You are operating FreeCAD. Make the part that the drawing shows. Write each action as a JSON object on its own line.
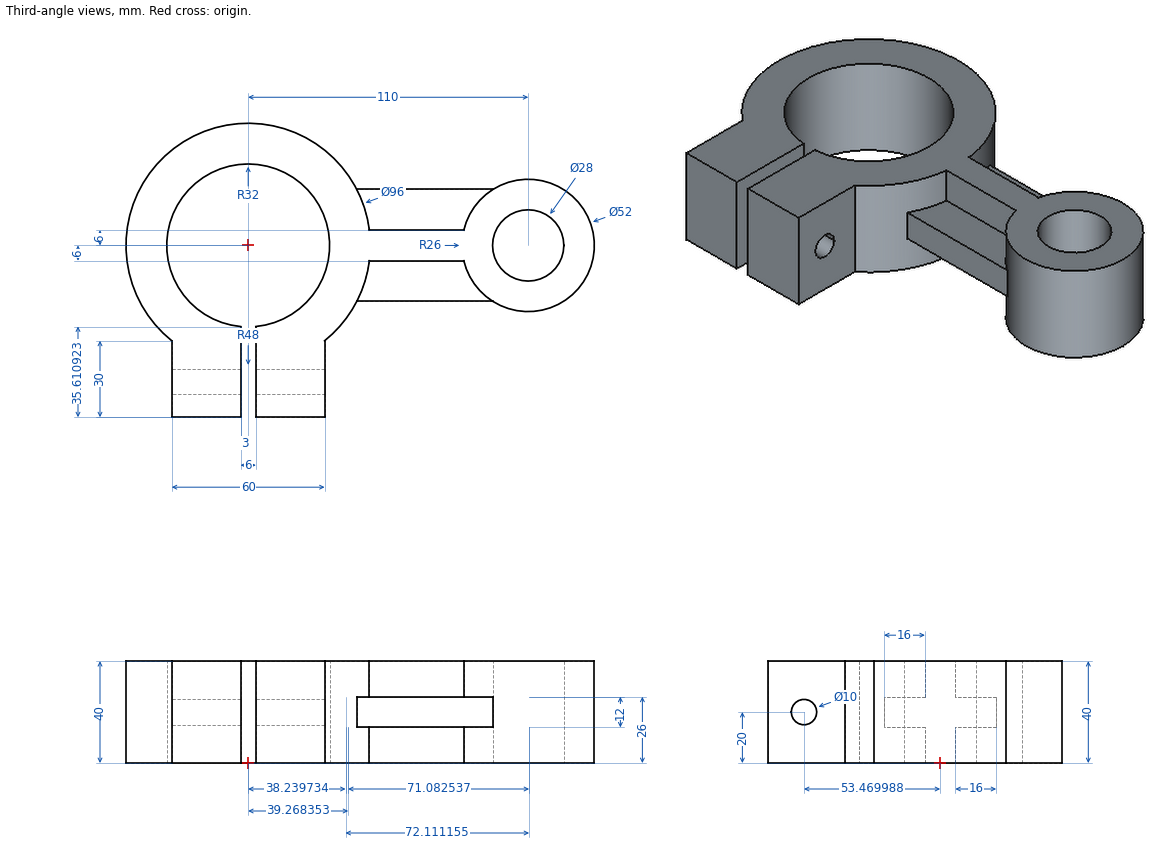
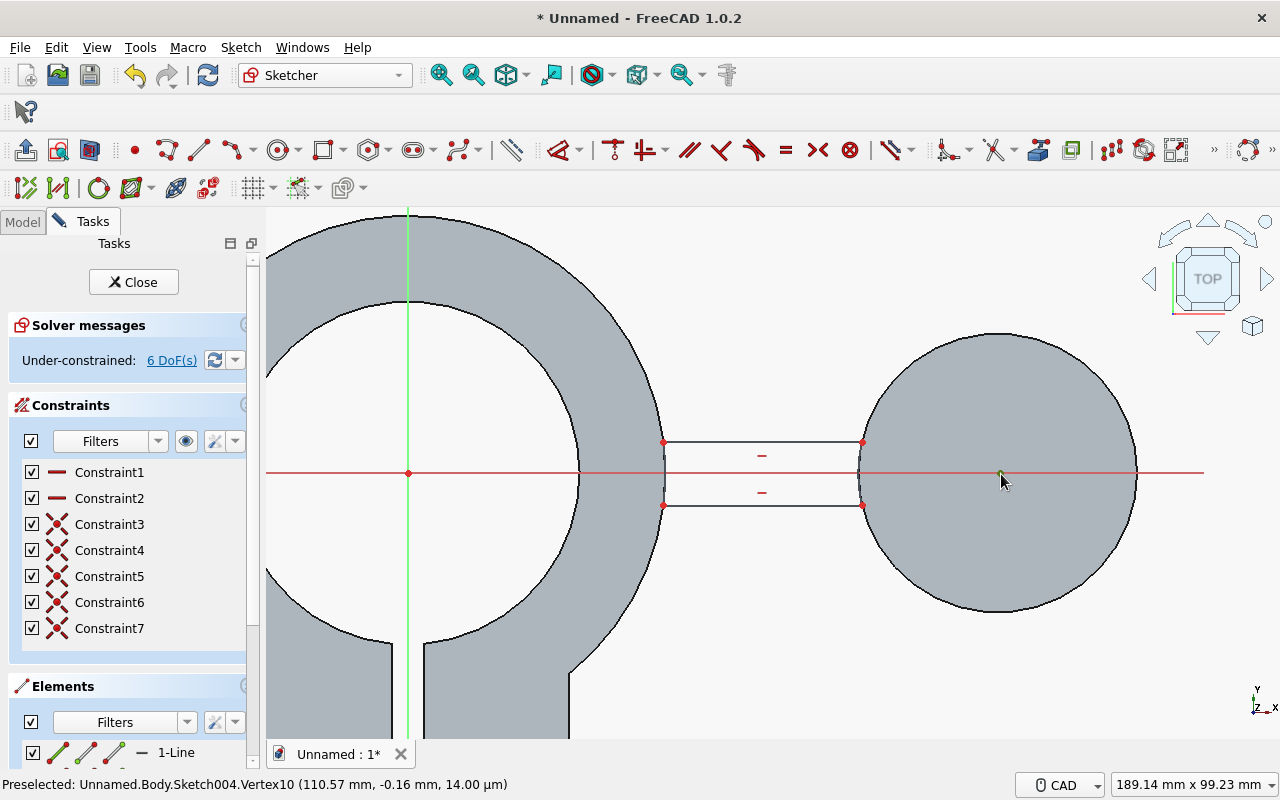
{"action": "left_click", "coordinate": [353, 473]}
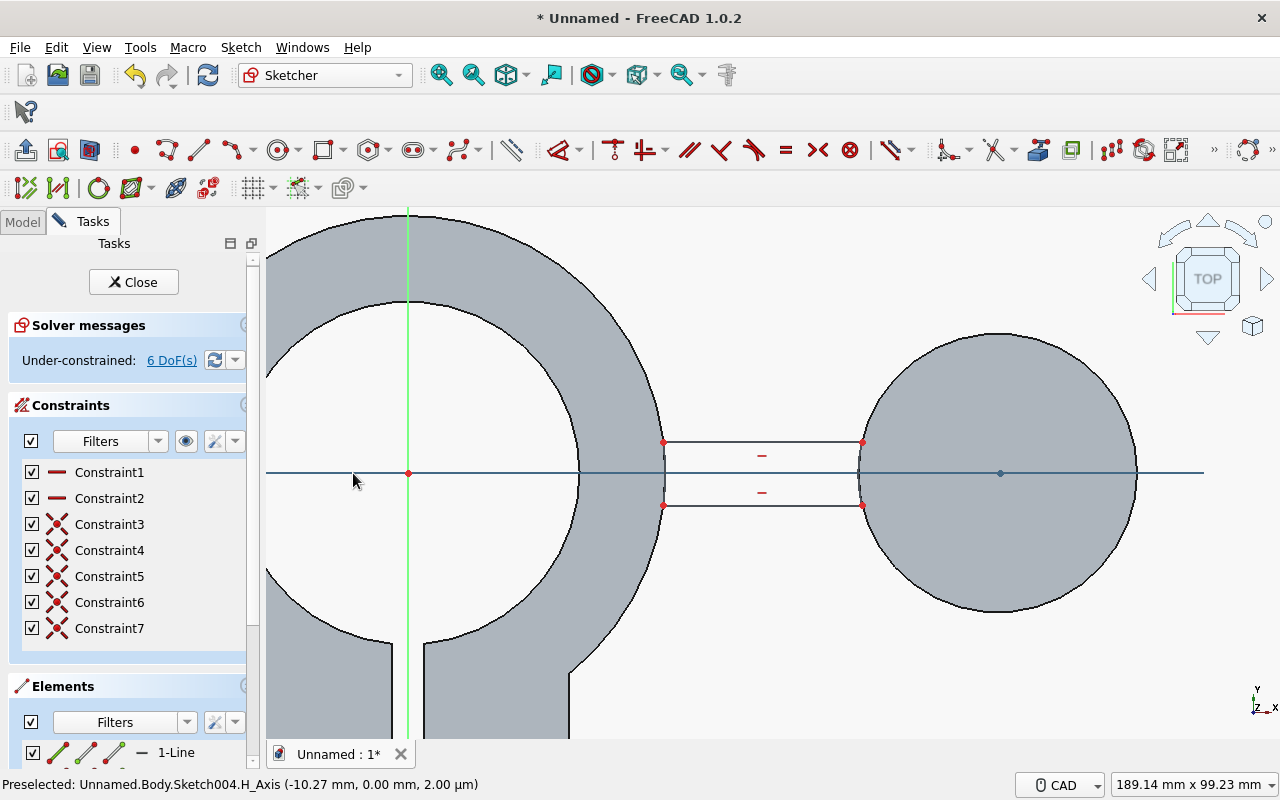
{"action": "left_click", "coordinate": [614, 150]}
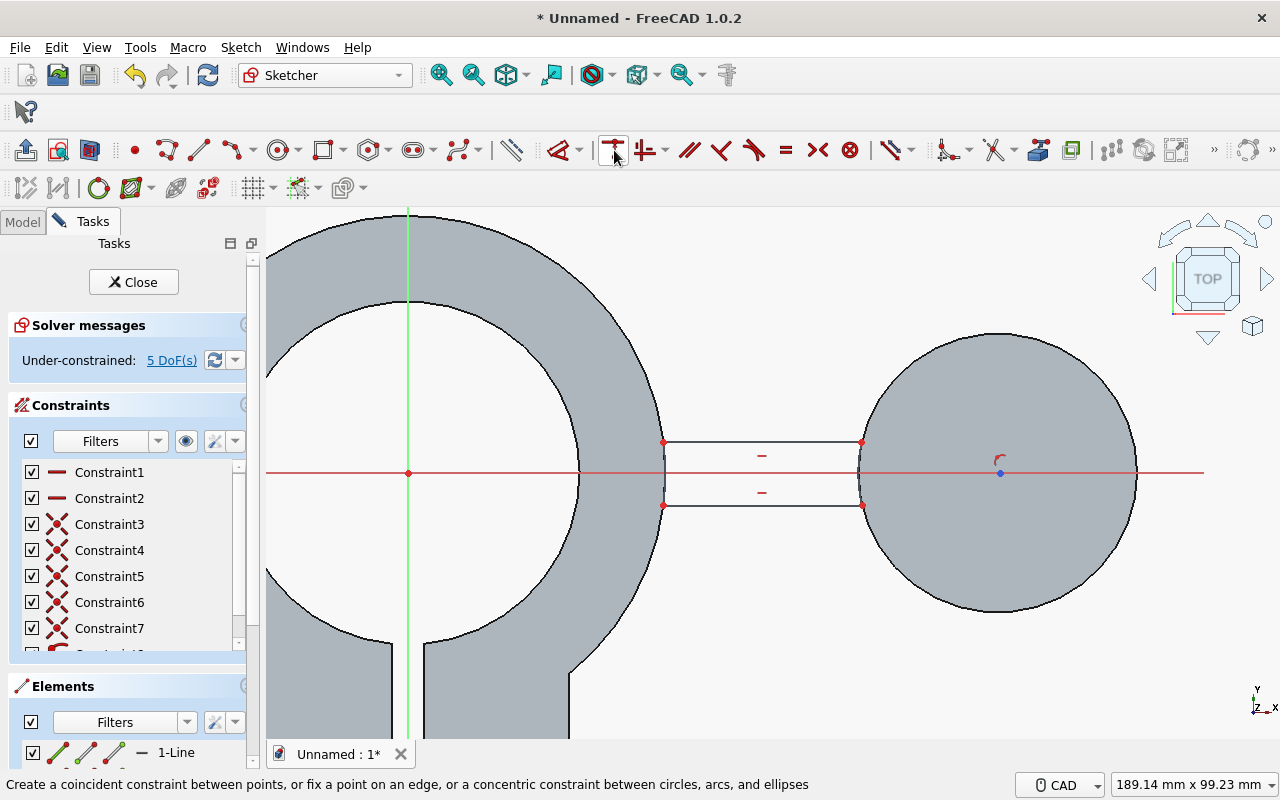
{"action": "left_click", "coordinate": [558, 150]}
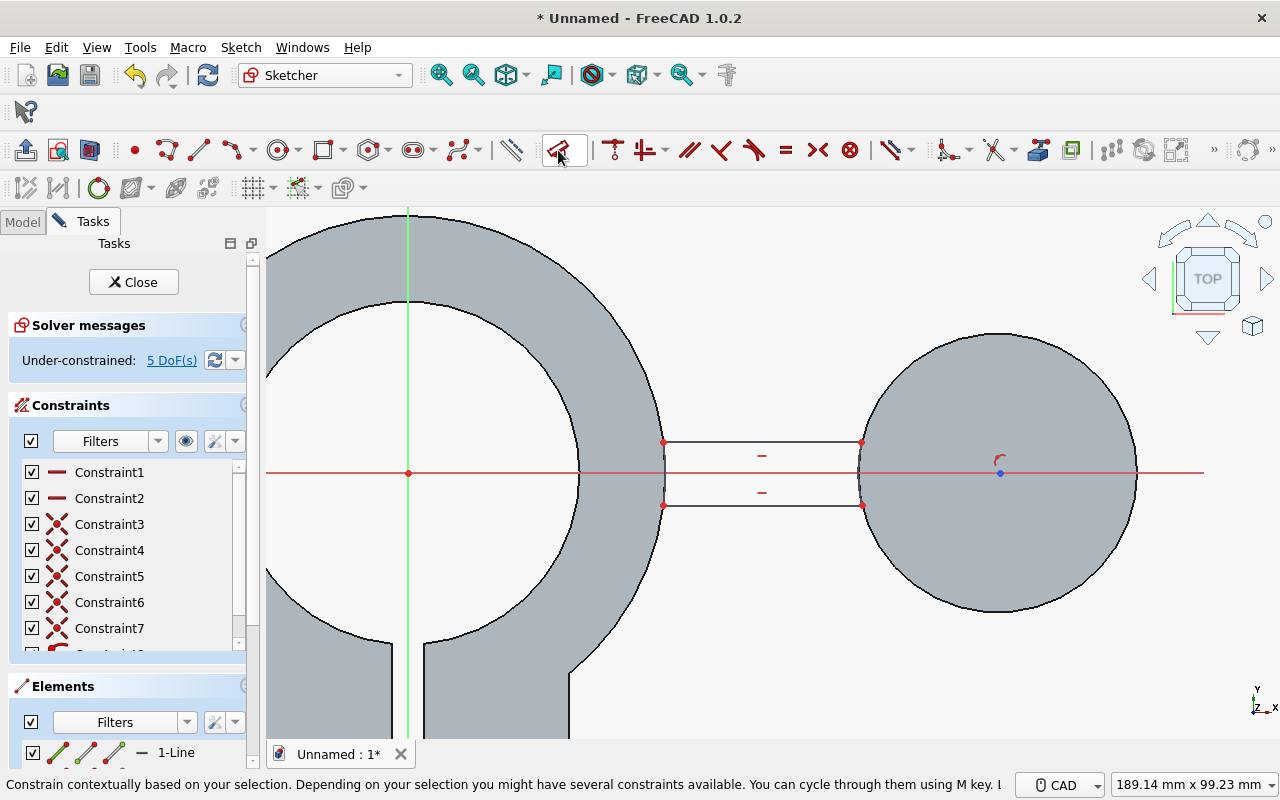
{"action": "left_click", "coordinate": [665, 487]}
{"action": "left_click", "coordinate": [697, 489]}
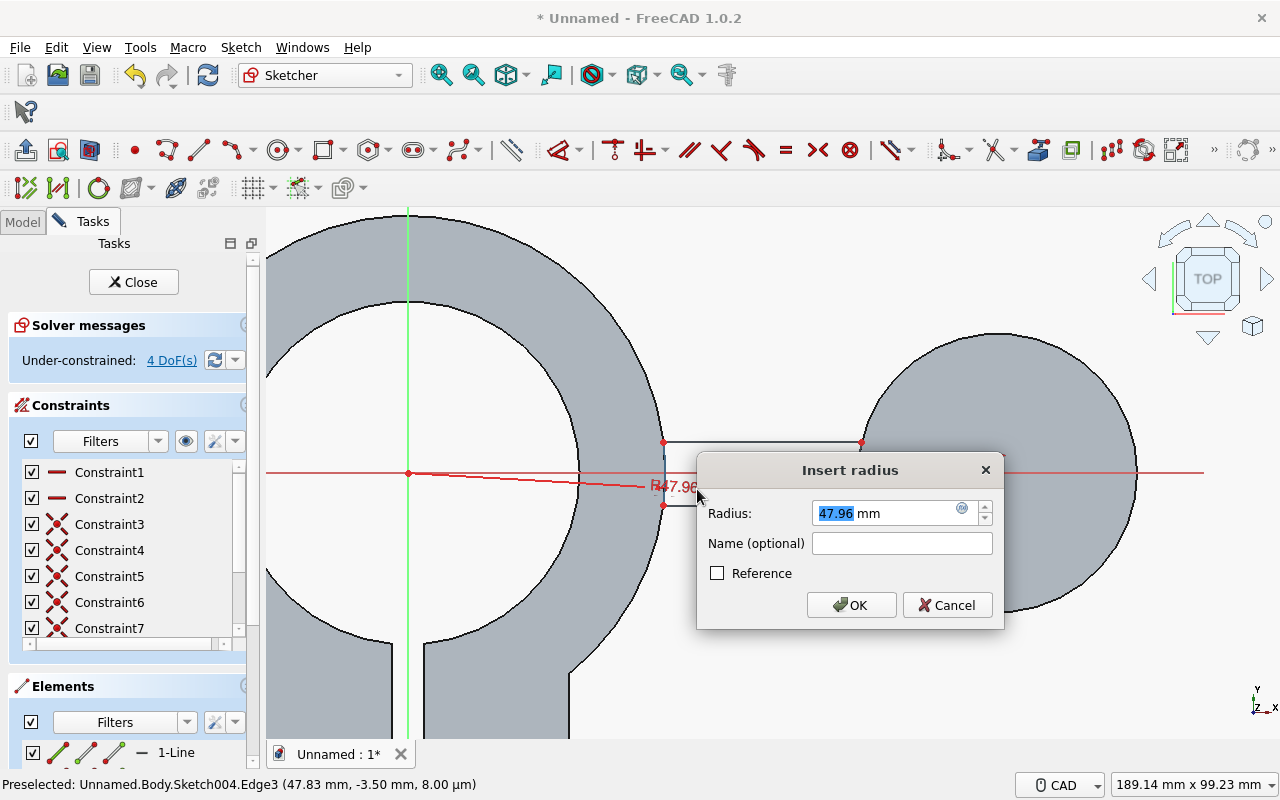
{"action": "type", "text": "48"}
{"action": "key", "text": "Return"}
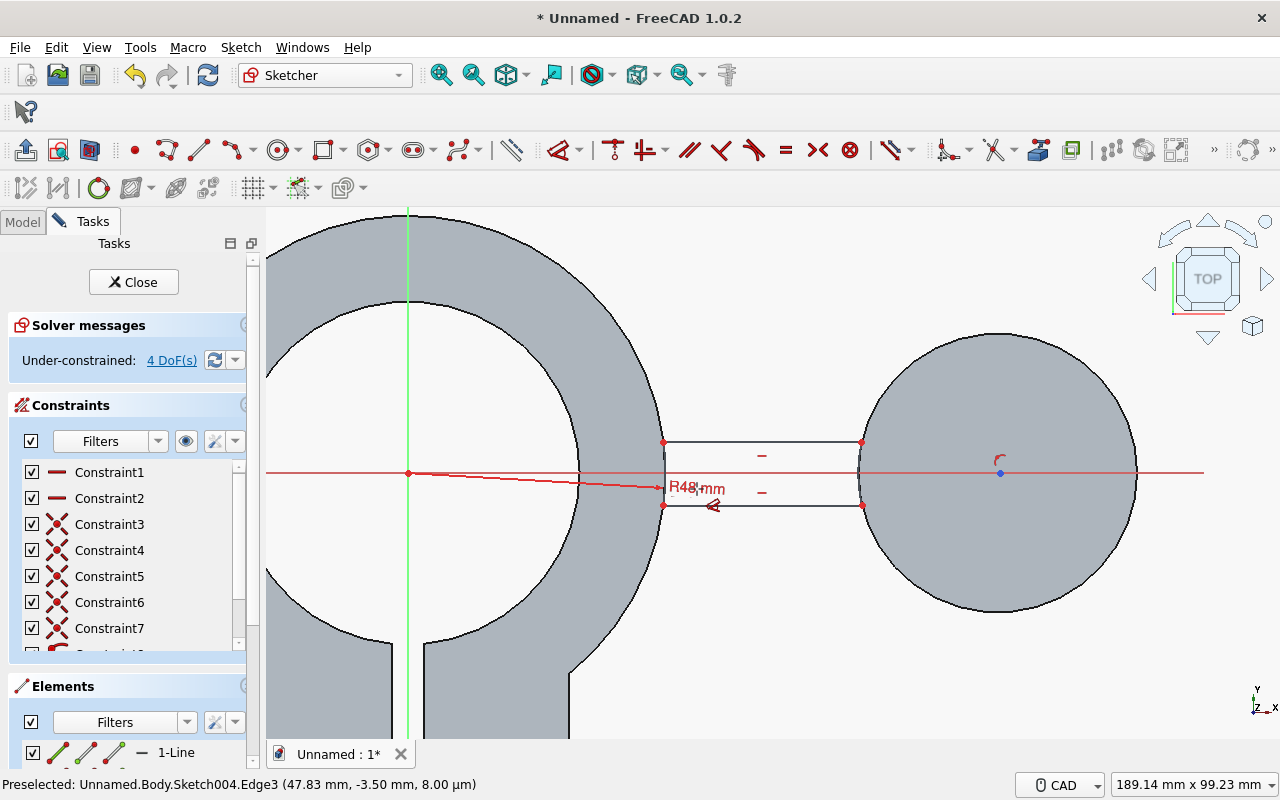
{"action": "left_click", "coordinate": [859, 461]}
{"action": "left_click", "coordinate": [827, 458]}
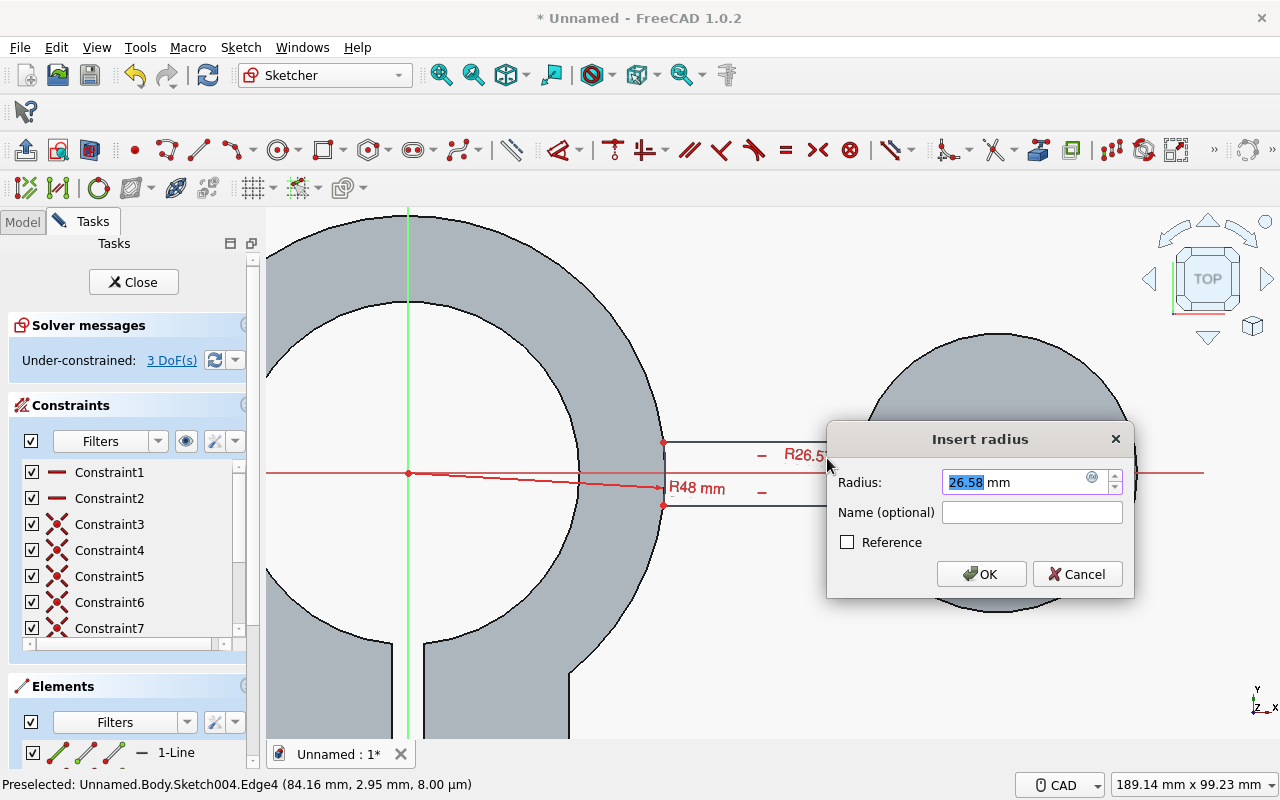
{"action": "type", "text": "26"}
{"action": "key", "text": "Return"}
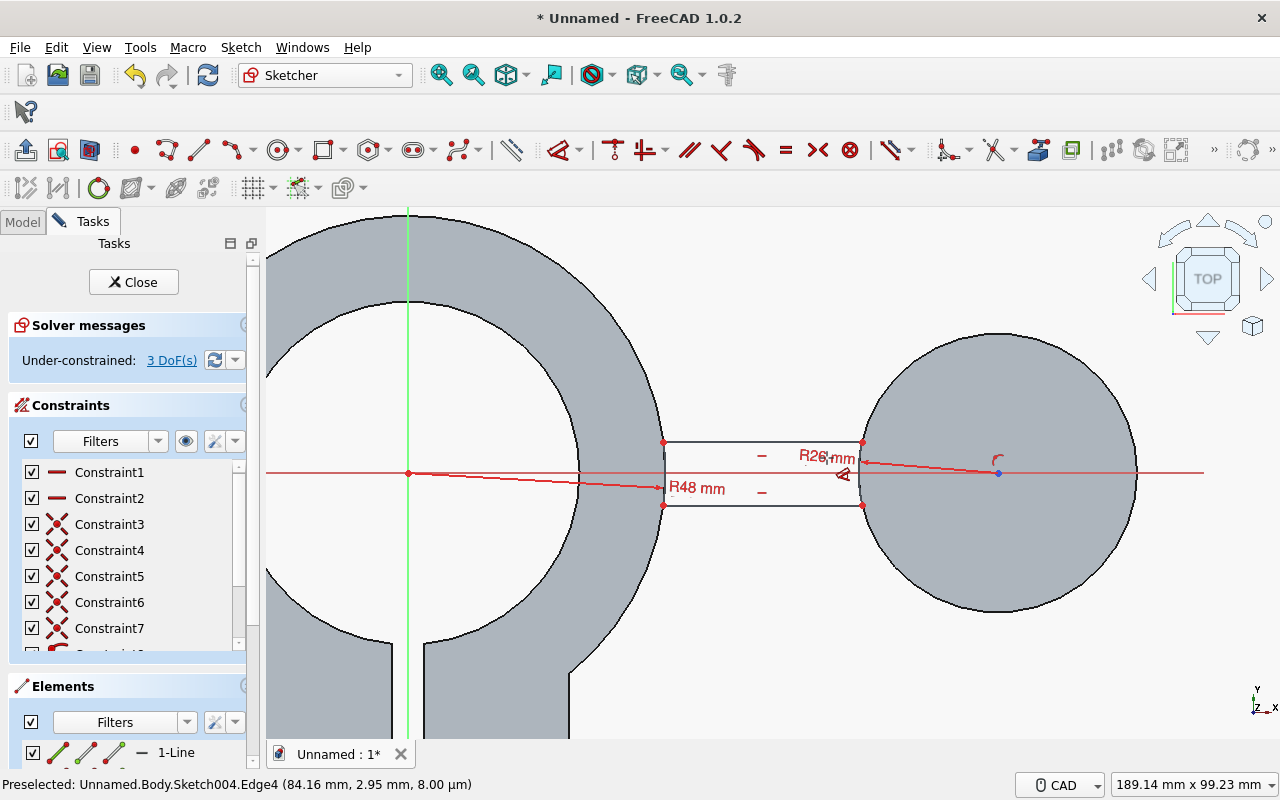
{"action": "scroll", "coordinate": [862, 442], "scroll_direction": "up", "scroll_amount": 2}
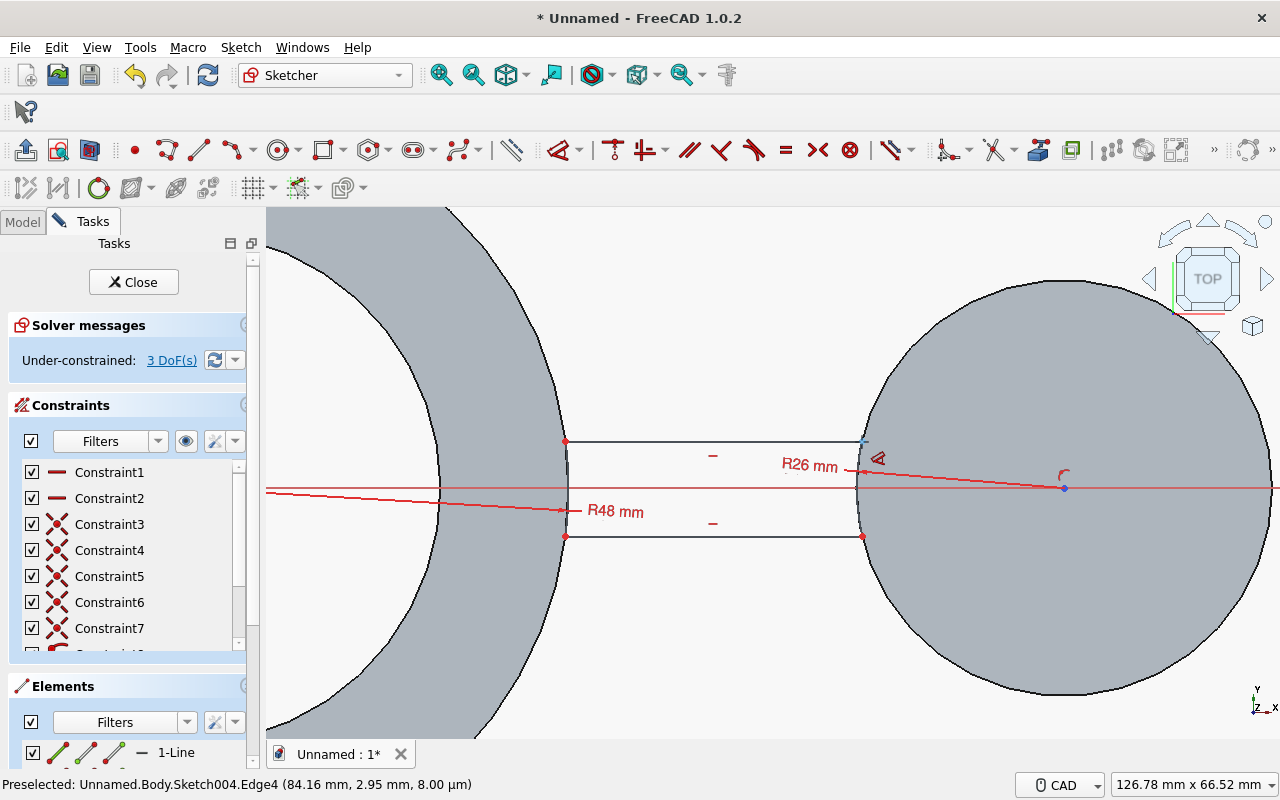
{"action": "left_click", "coordinate": [862, 442]}
{"action": "left_click", "coordinate": [896, 465]}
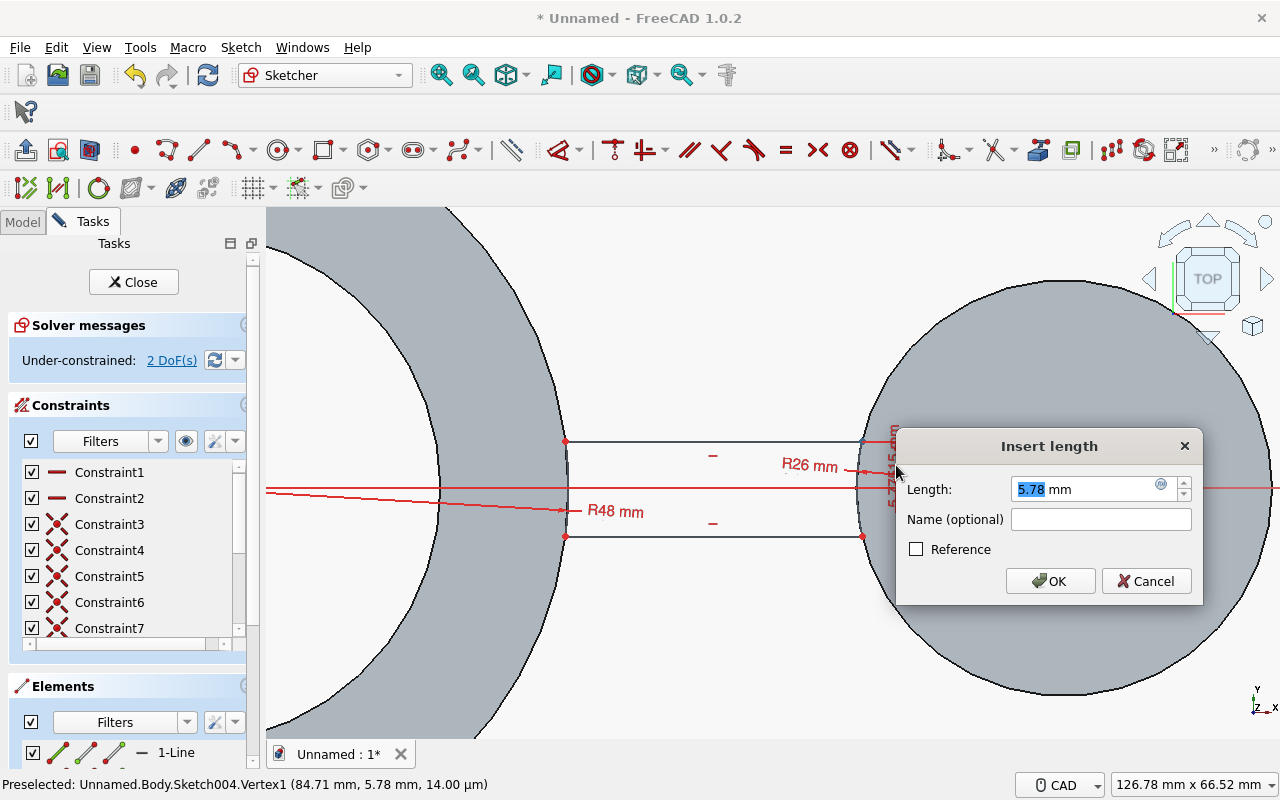
{"action": "type", "text": "6"}
{"action": "key", "text": "Return"}